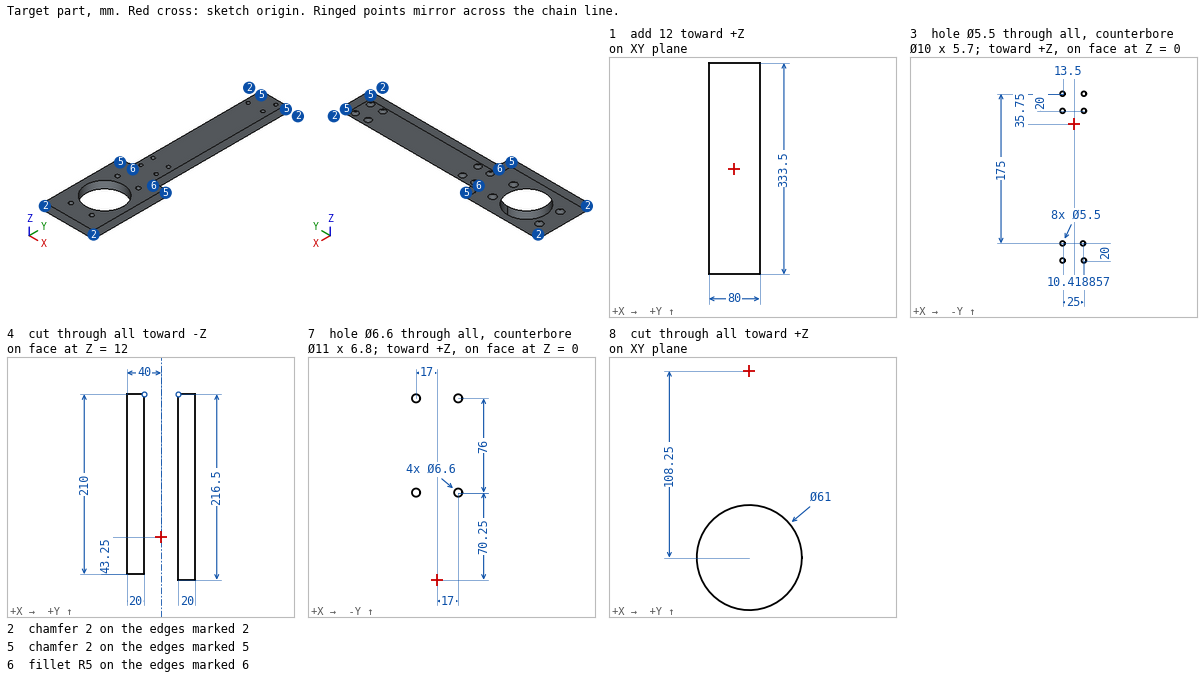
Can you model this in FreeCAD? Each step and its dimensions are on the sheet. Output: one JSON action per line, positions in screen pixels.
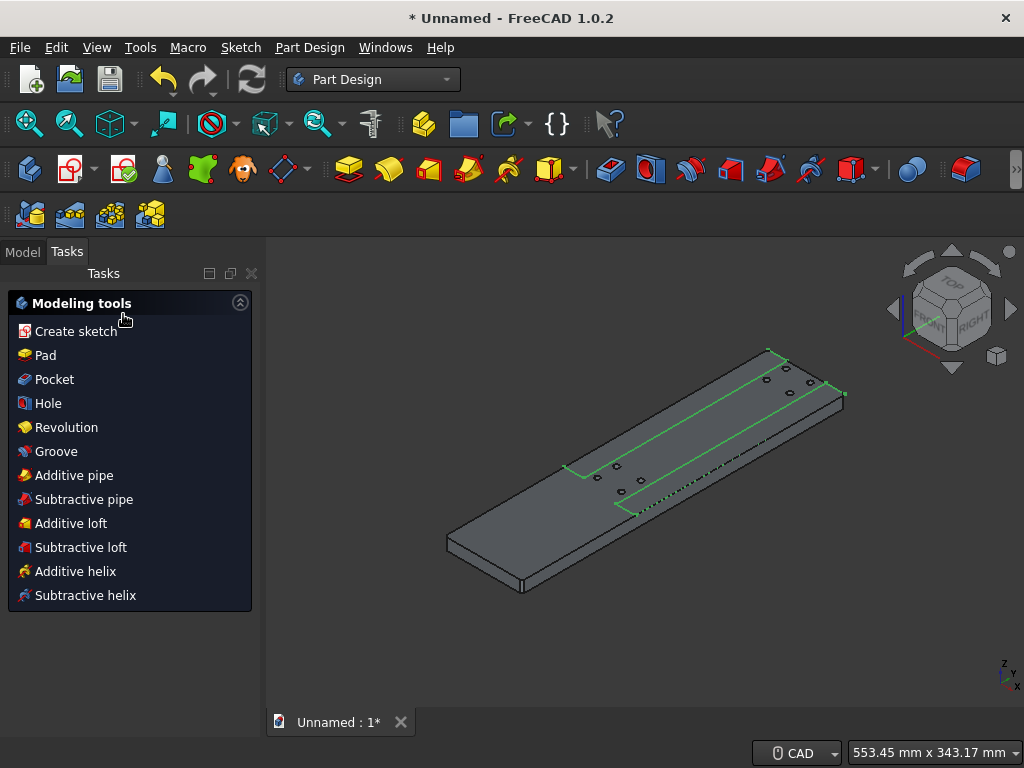
{"action": "left_click", "coordinate": [612, 170]}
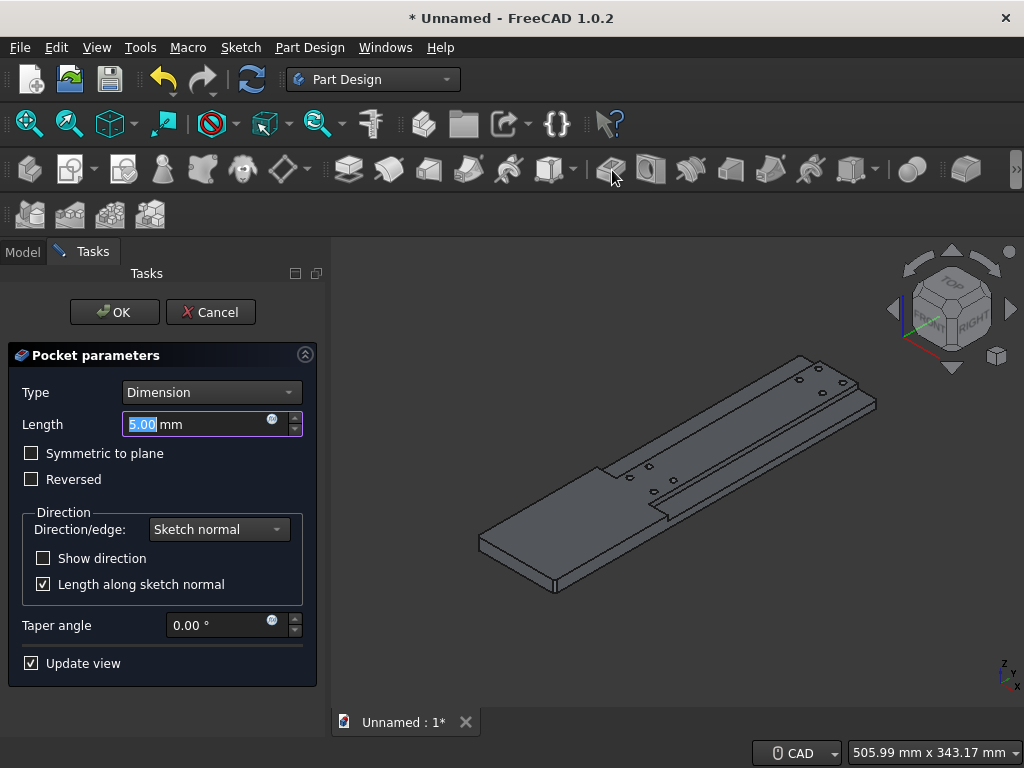
{"action": "left_click", "coordinate": [212, 392]}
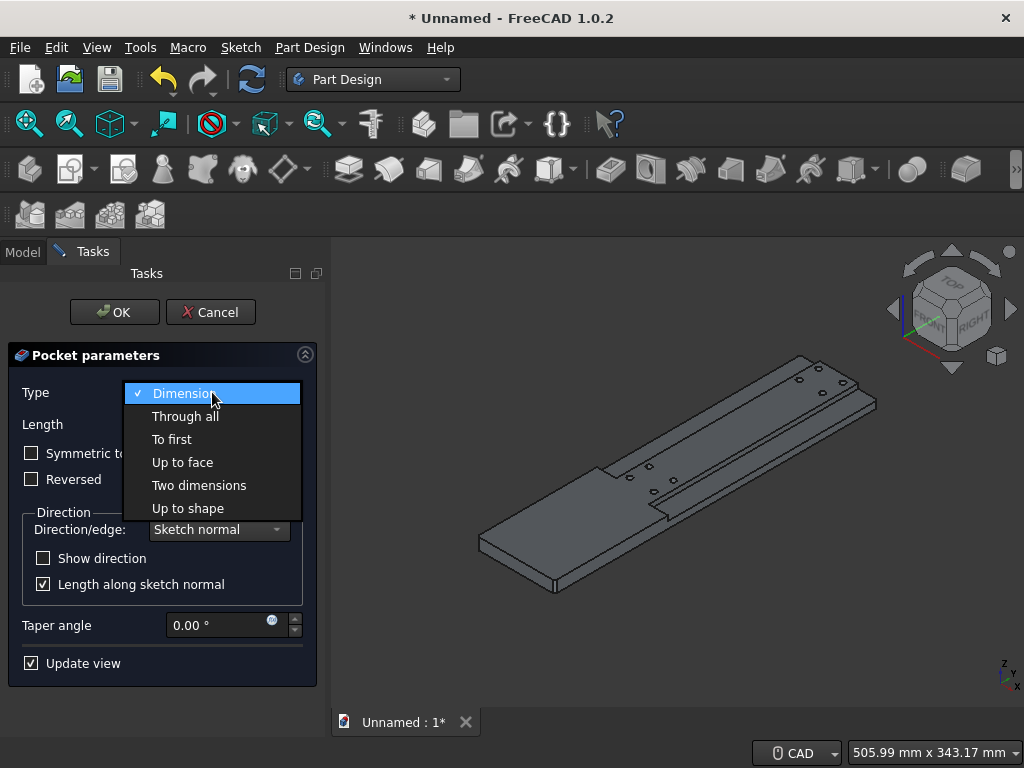
{"action": "left_click", "coordinate": [212, 416]}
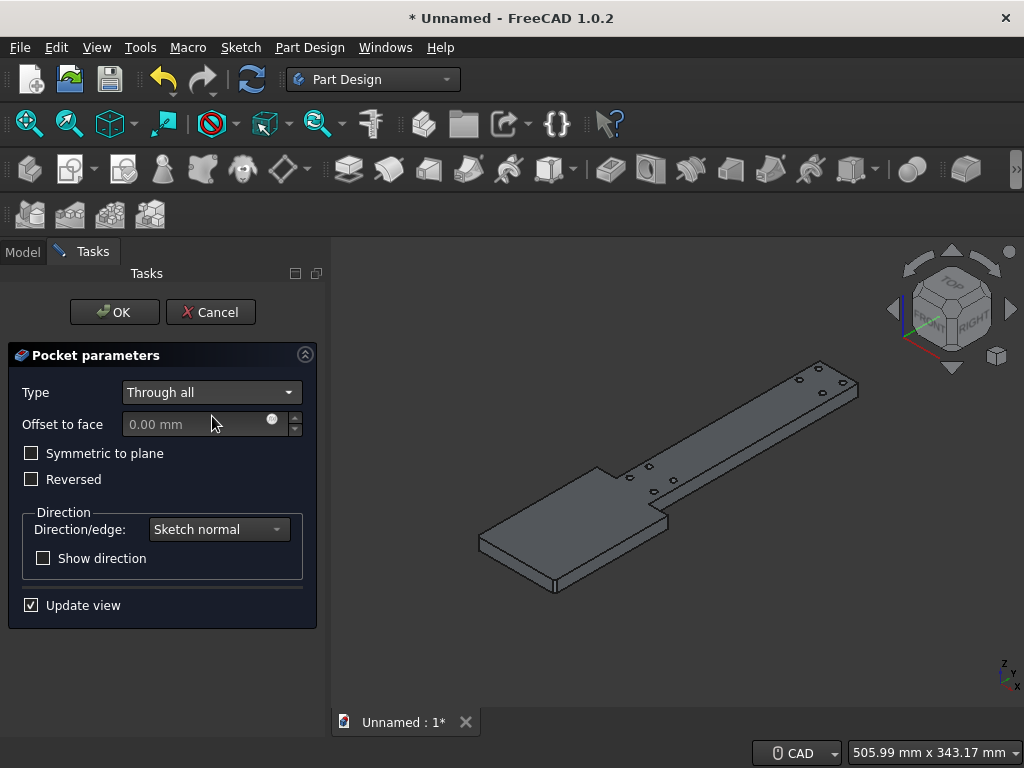
{"action": "left_click", "coordinate": [115, 312]}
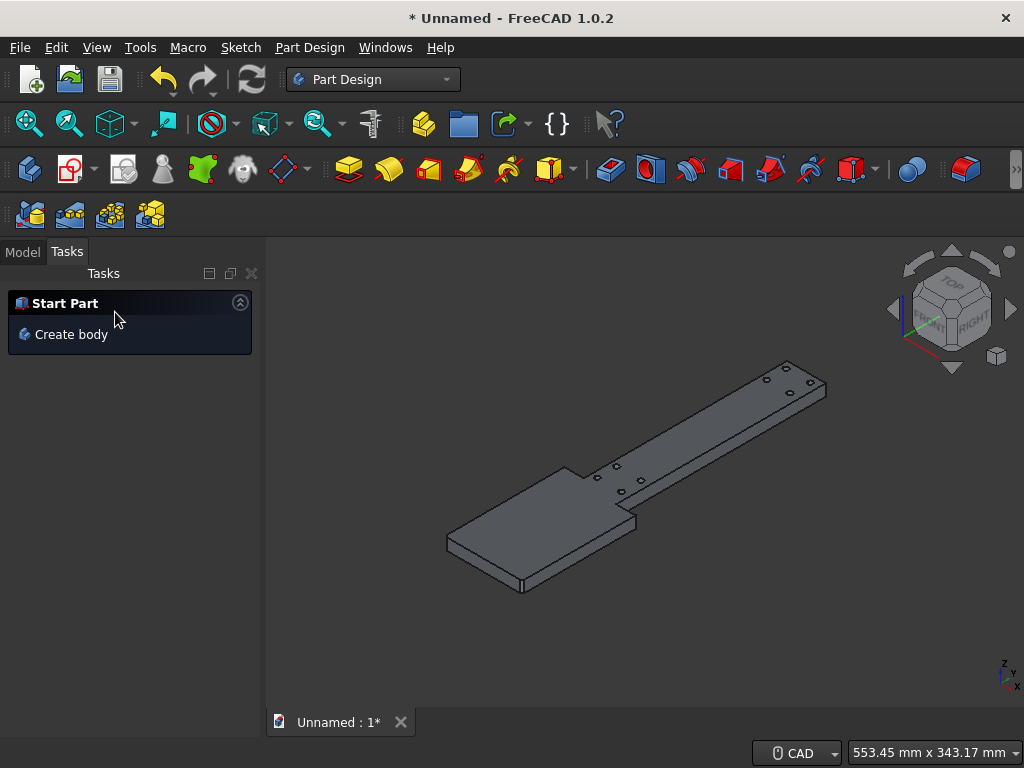
{"action": "scroll", "coordinate": [564, 473], "scroll_direction": "up", "scroll_amount": 5}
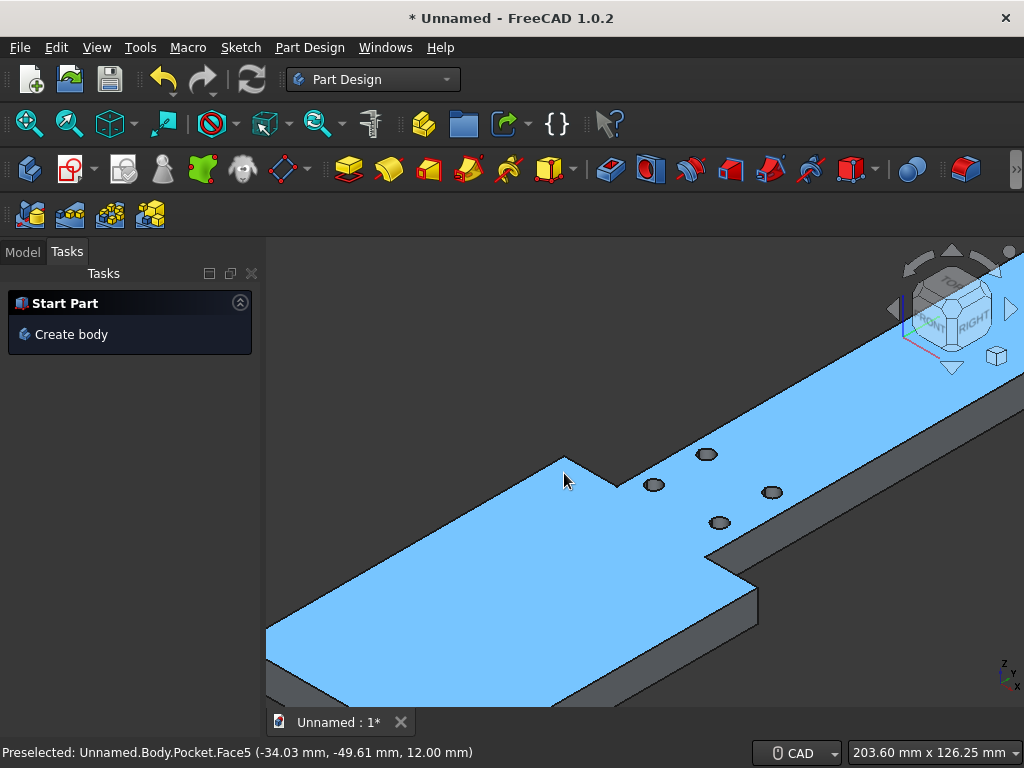
{"action": "key", "text": "v f"}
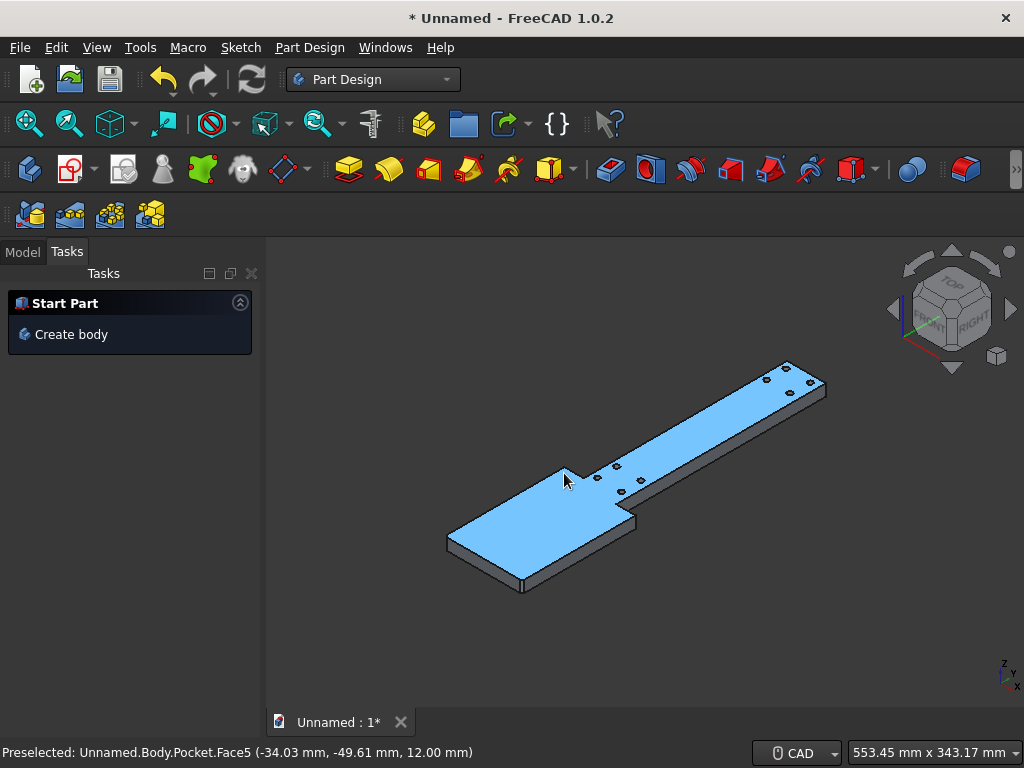
{"action": "key", "text": "2"}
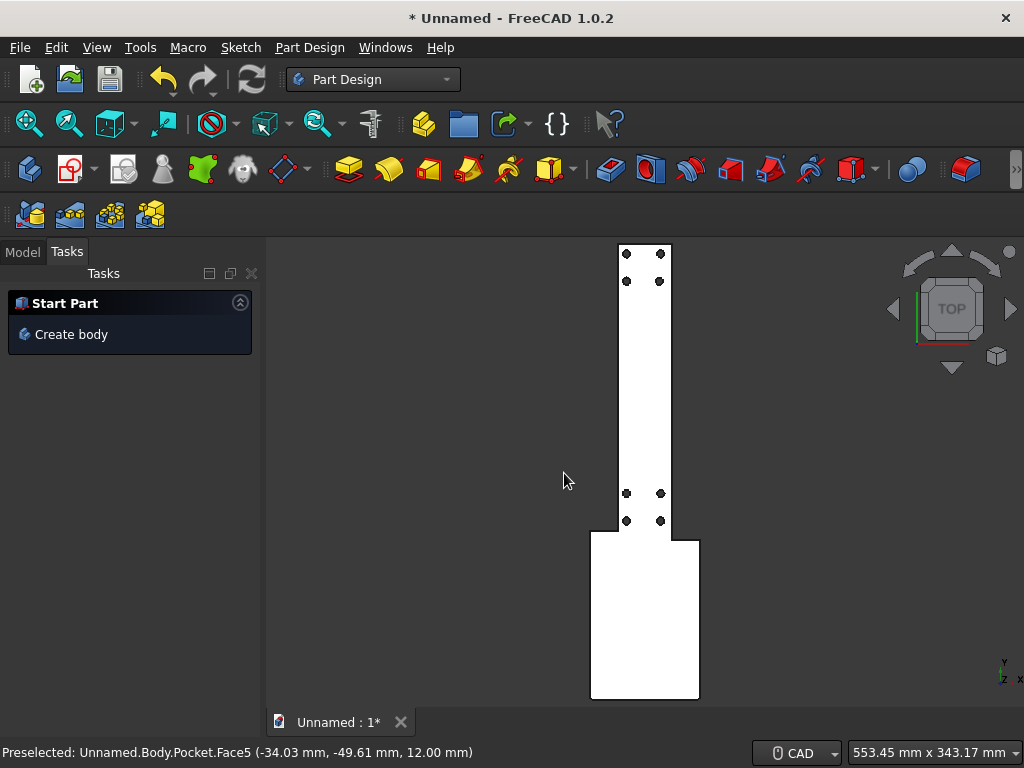
{"action": "scroll", "coordinate": [590, 530], "scroll_direction": "up", "scroll_amount": 5}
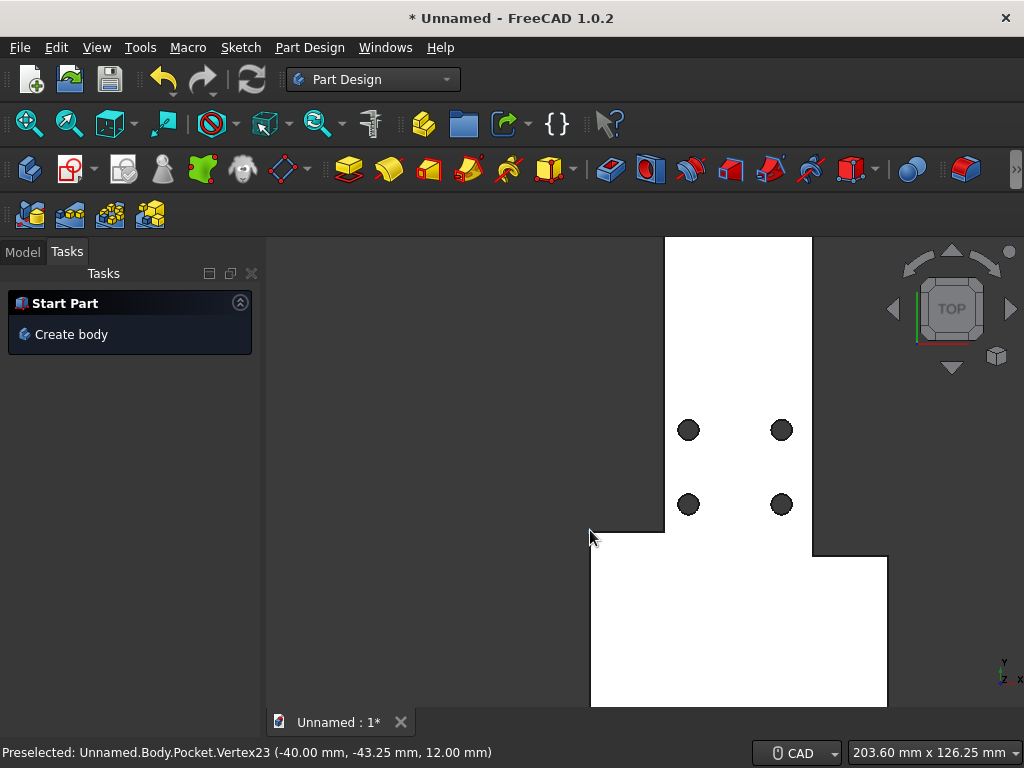
{"action": "key", "text": "v f"}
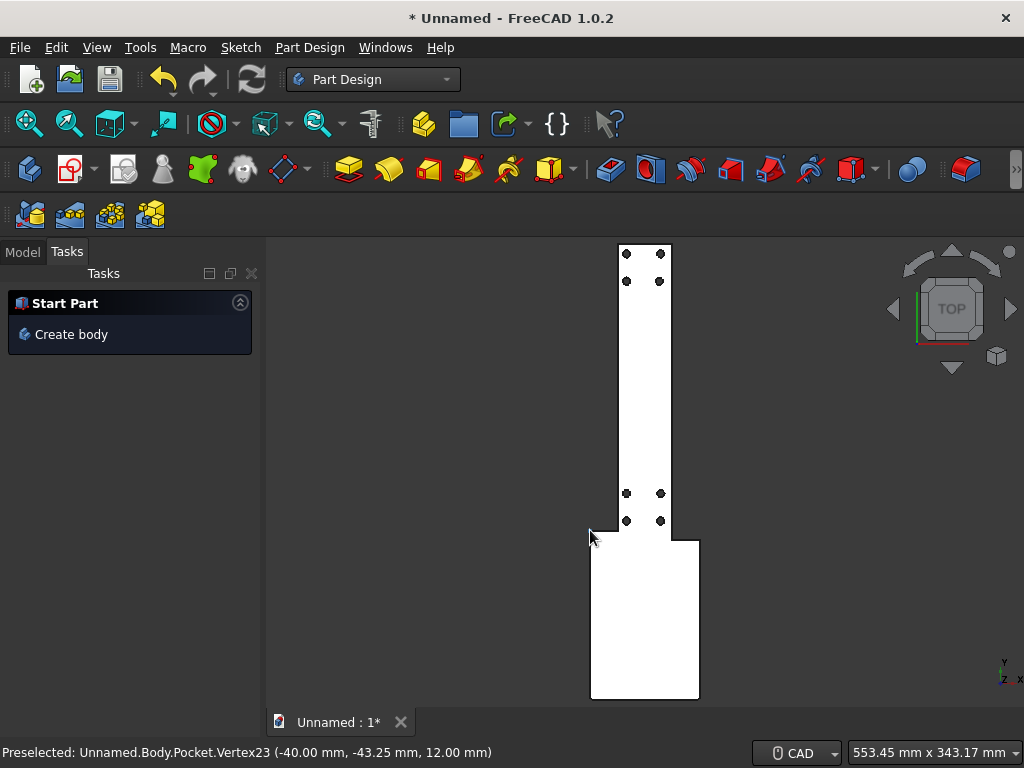
{"action": "key", "text": "0"}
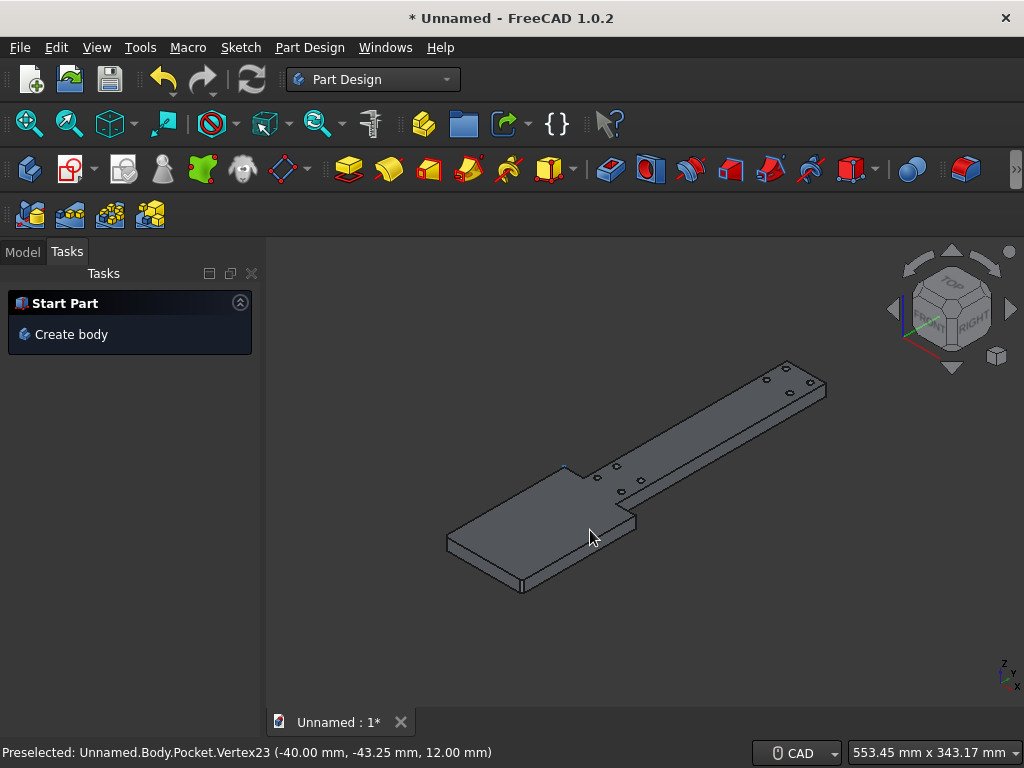
{"action": "scroll", "coordinate": [564, 473], "scroll_direction": "up", "scroll_amount": 5}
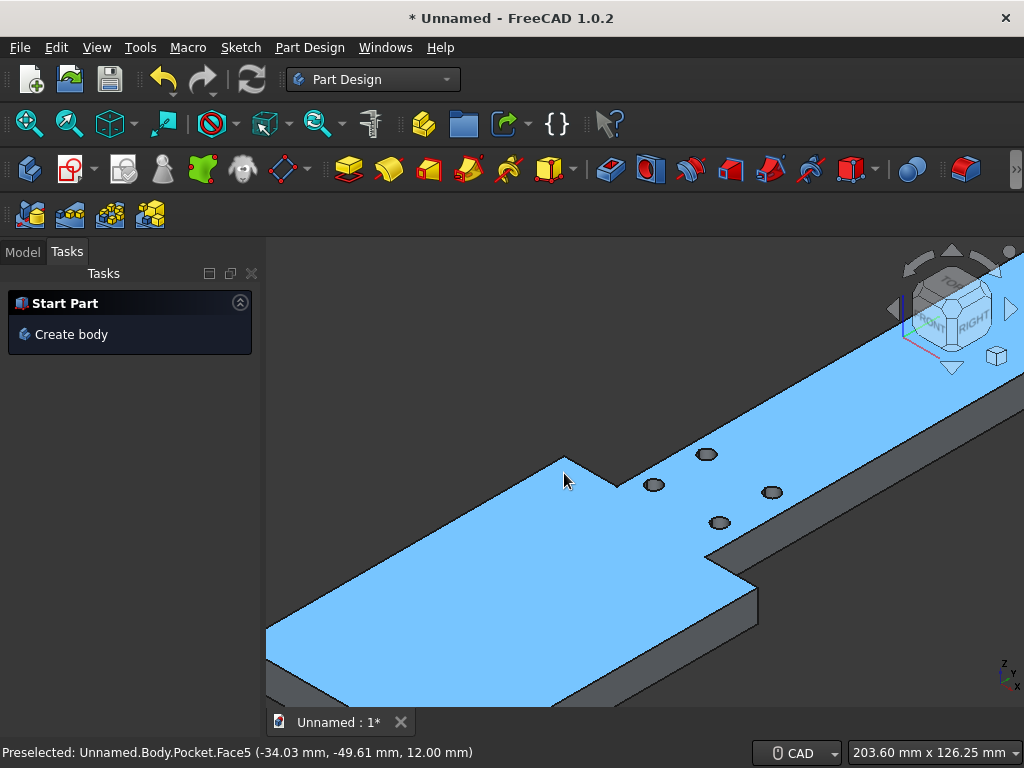
{"action": "key", "text": "v f"}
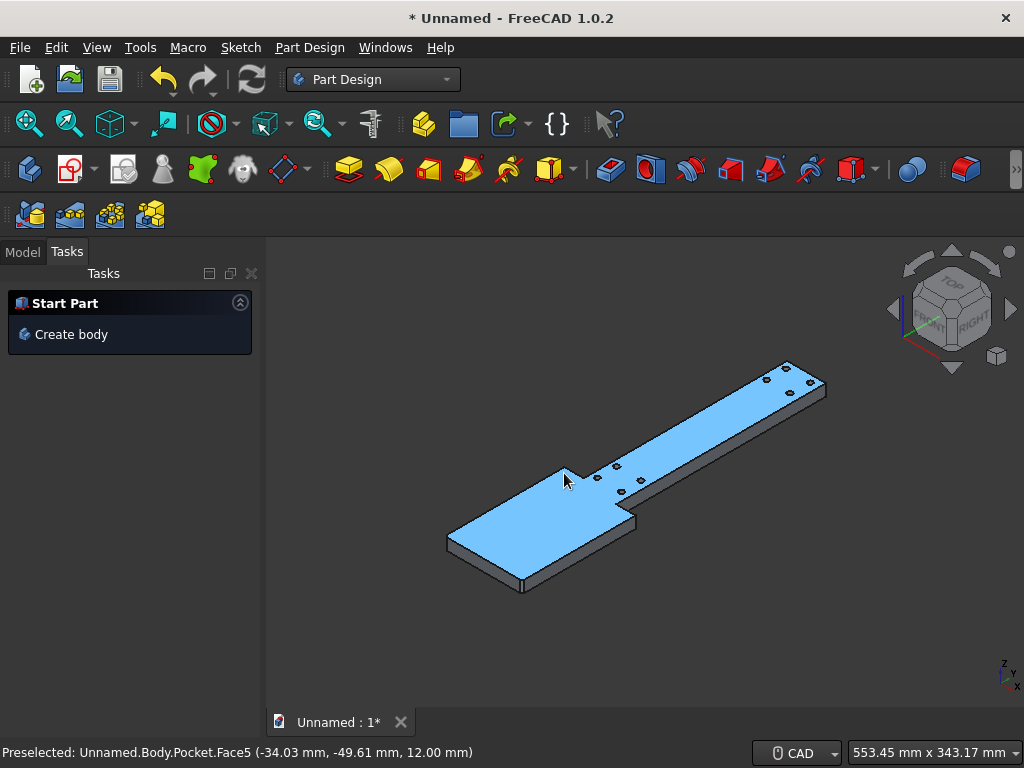
{"action": "key", "text": "1"}